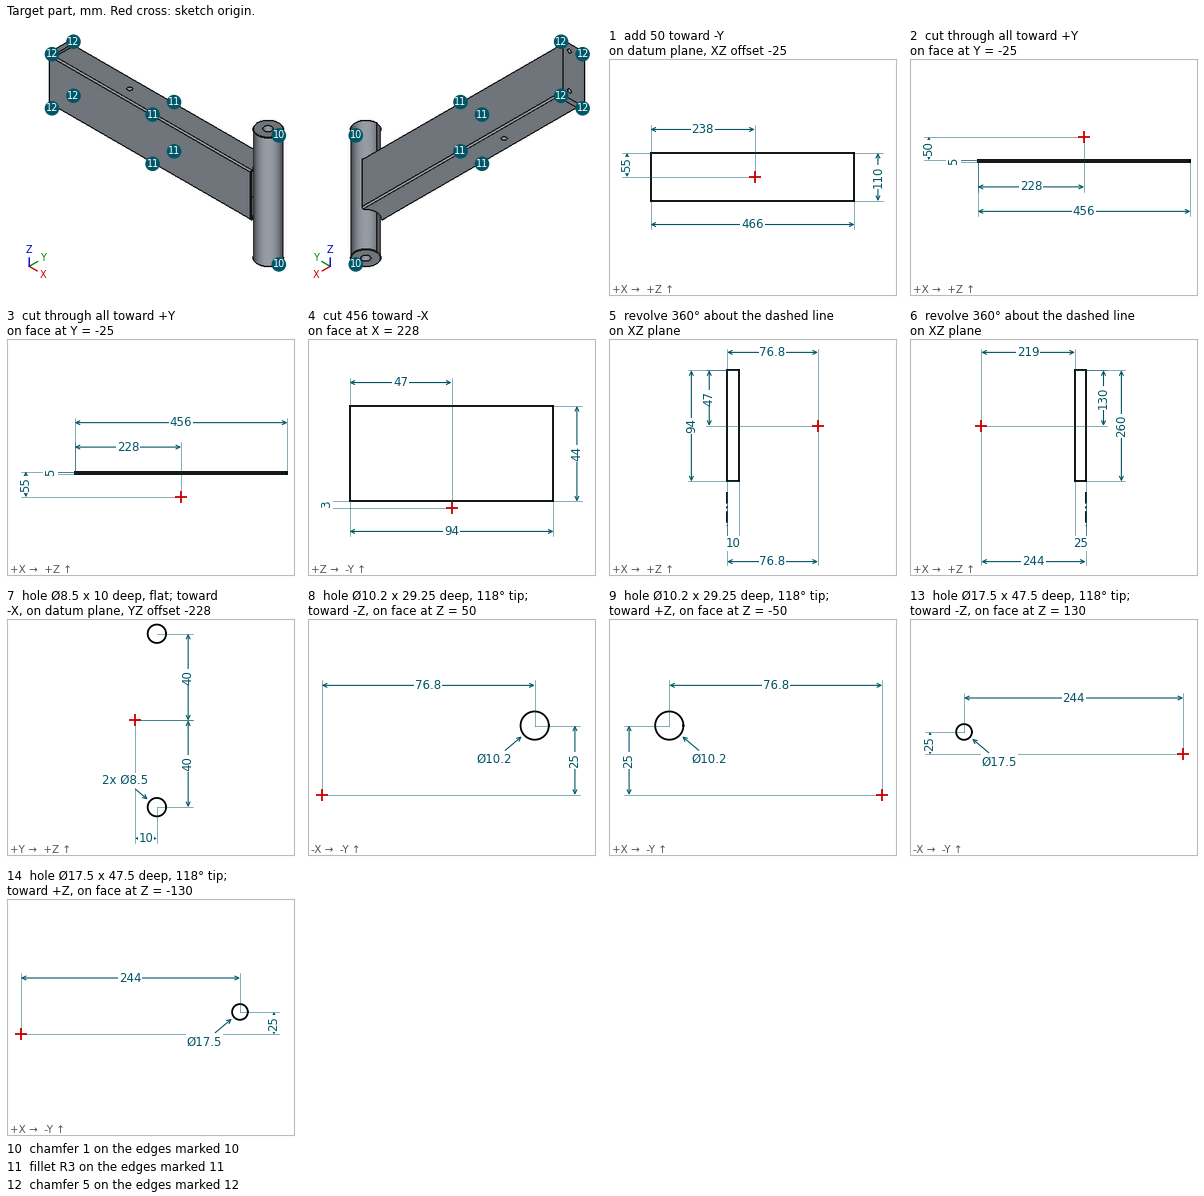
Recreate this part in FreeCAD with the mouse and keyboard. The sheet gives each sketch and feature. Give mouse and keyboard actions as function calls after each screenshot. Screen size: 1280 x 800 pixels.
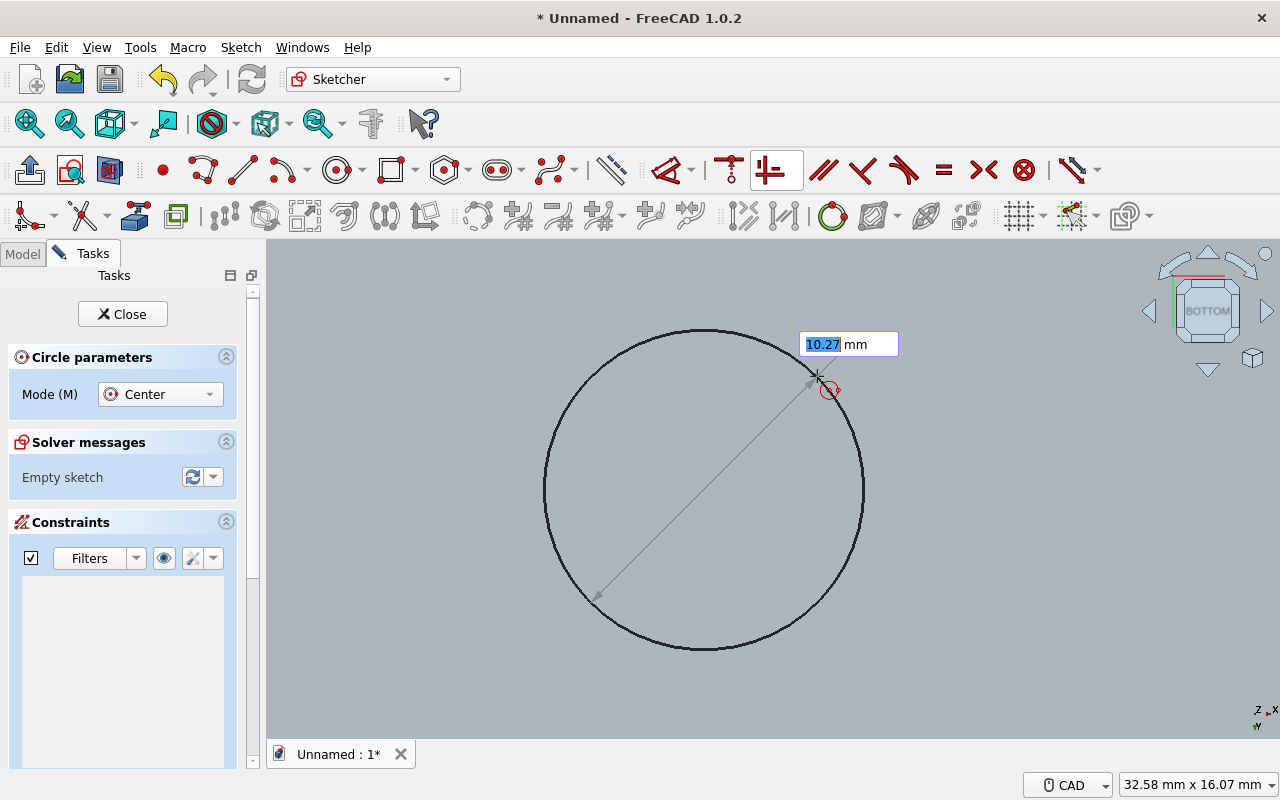
text(10.2)
key(Return)
key(Escape)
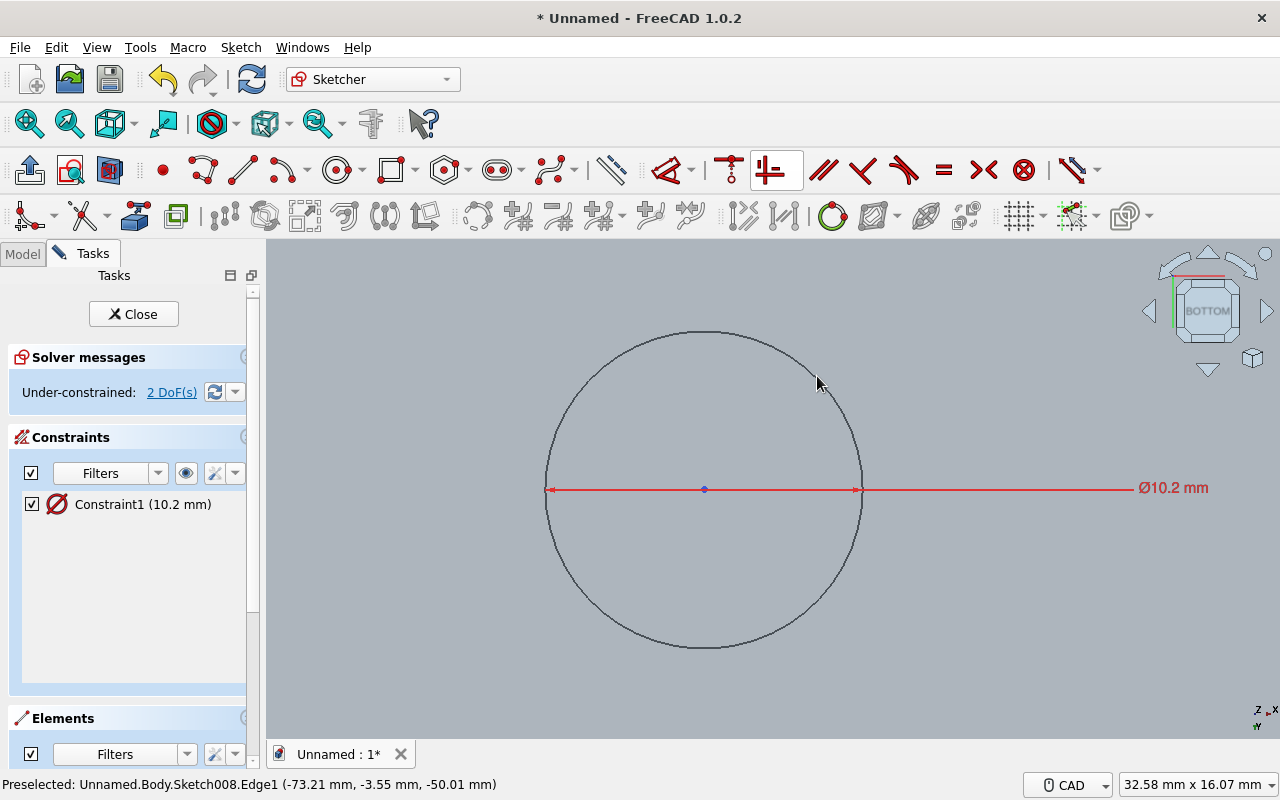
click(666, 170)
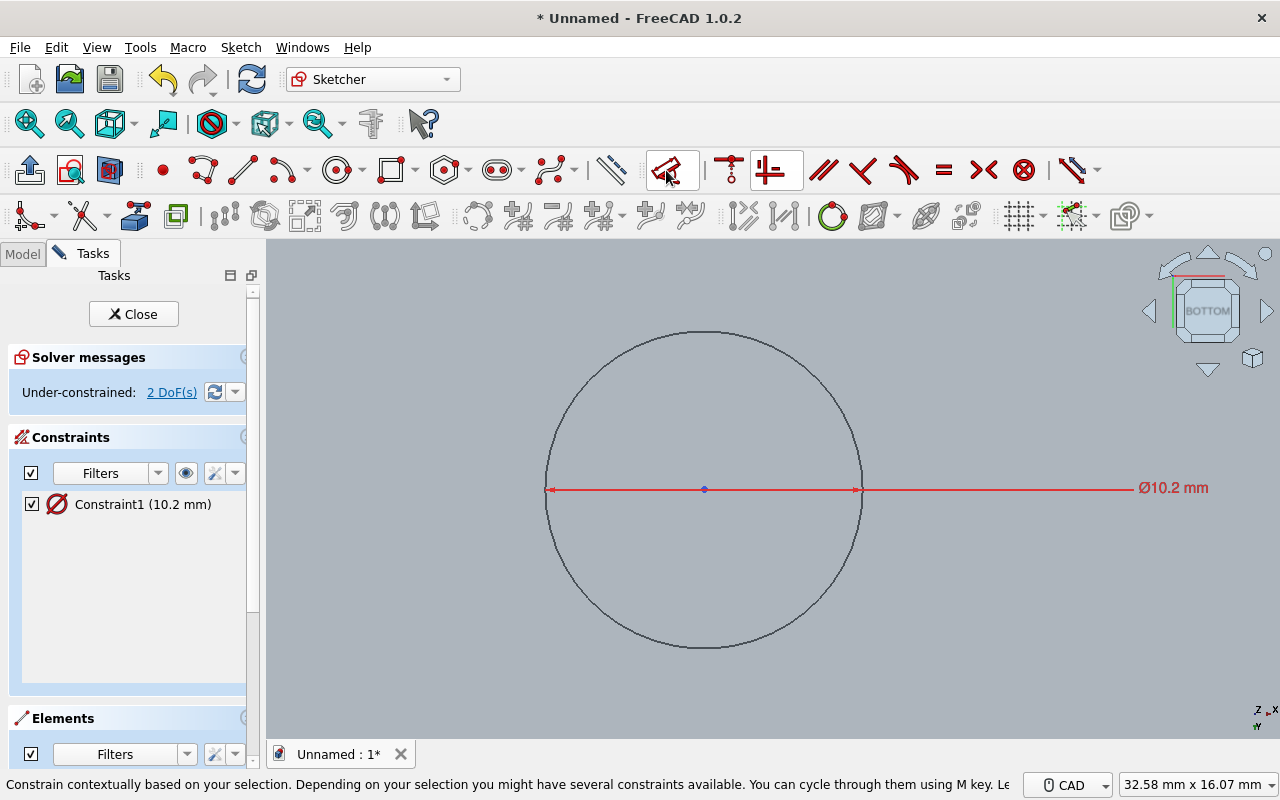
click(704, 490)
click(670, 601)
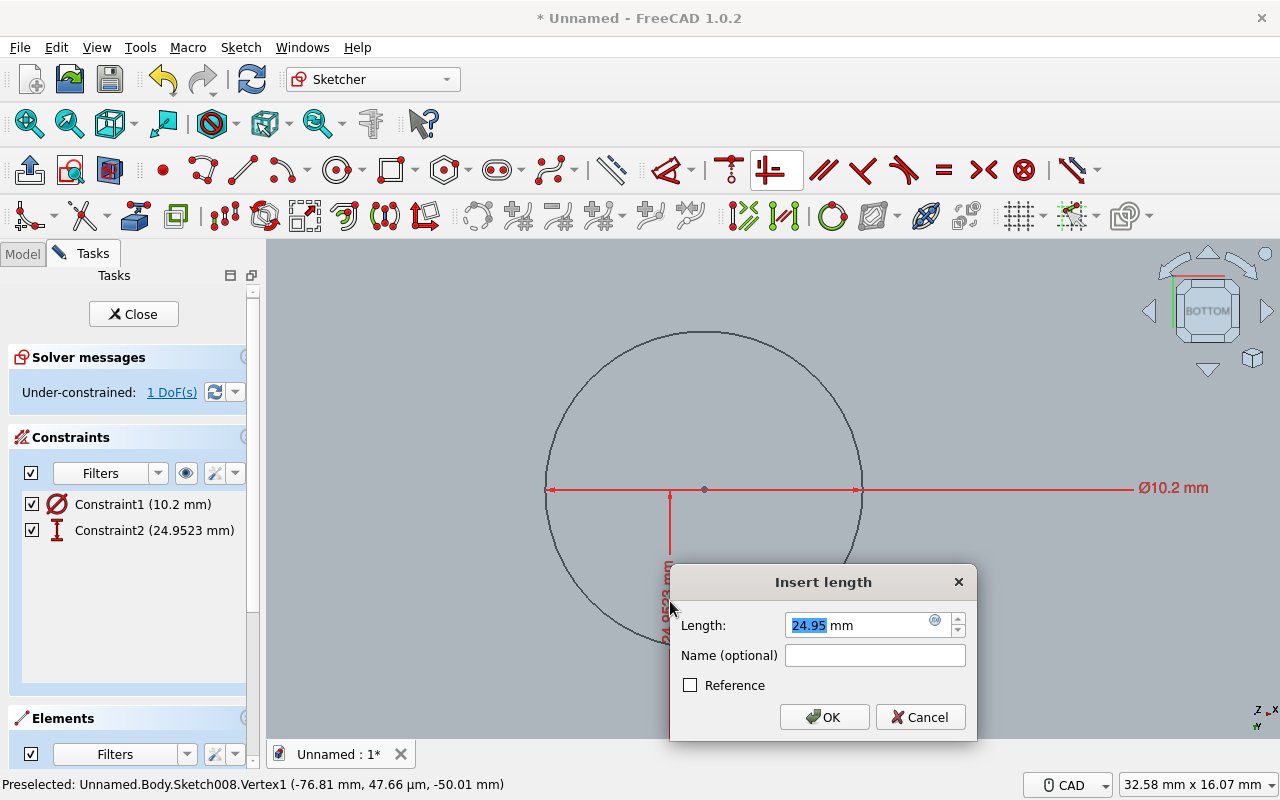
text(25)
key(Return)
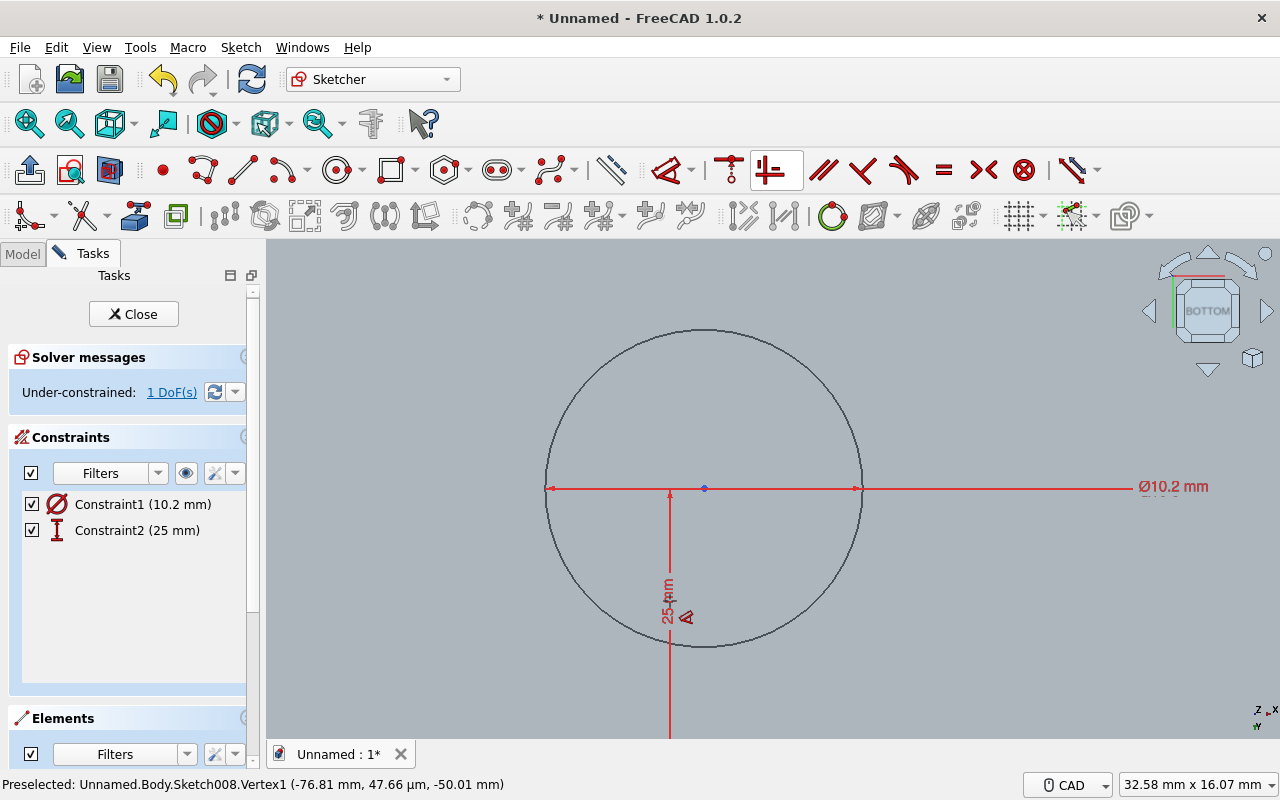
click(704, 489)
click(910, 455)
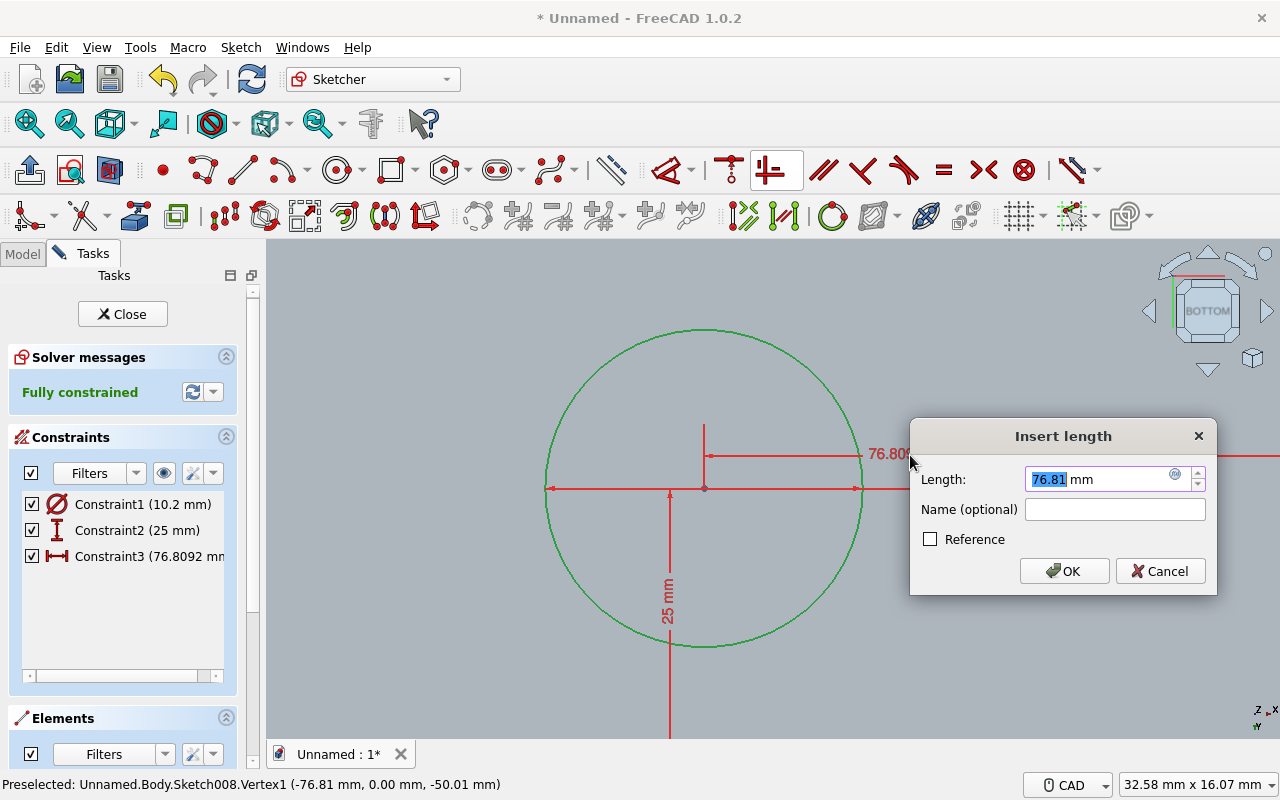
text(76.8)
key(Return)
key(Escape)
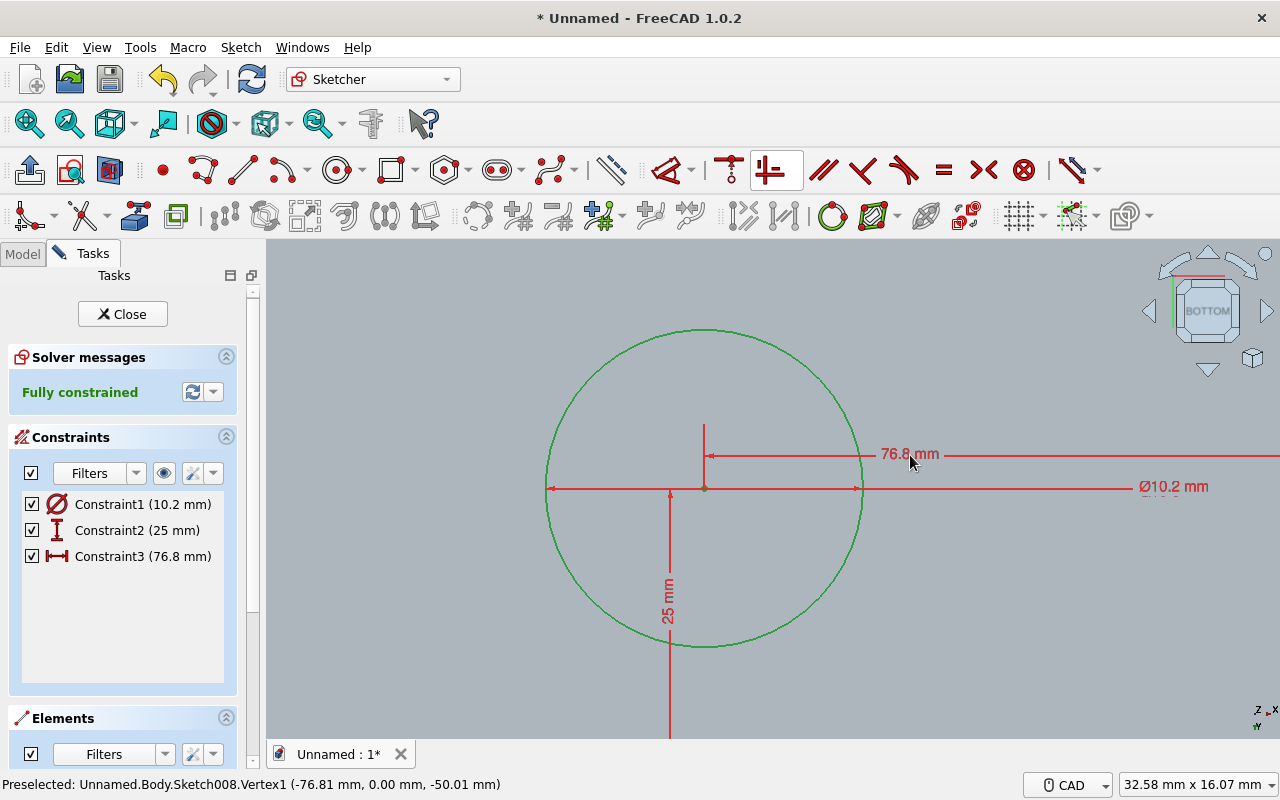
click(123, 314)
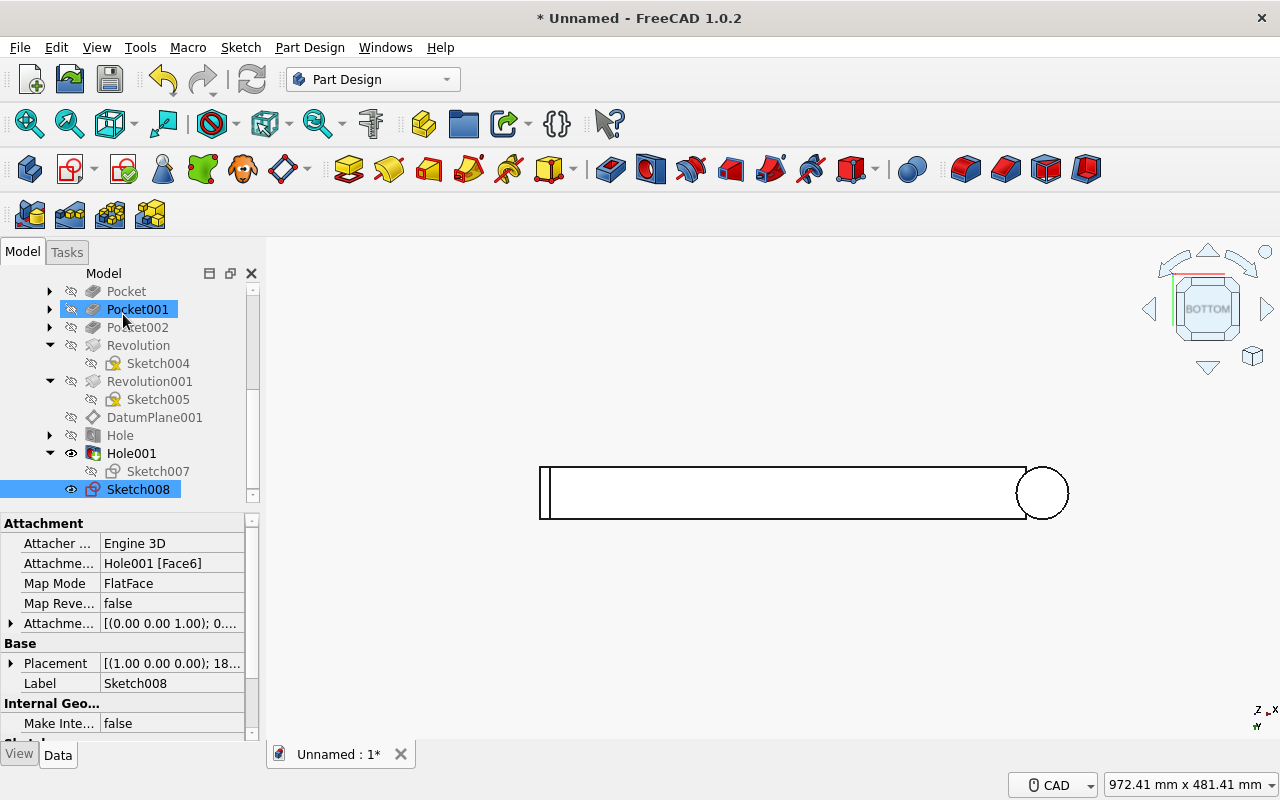
click(652, 170)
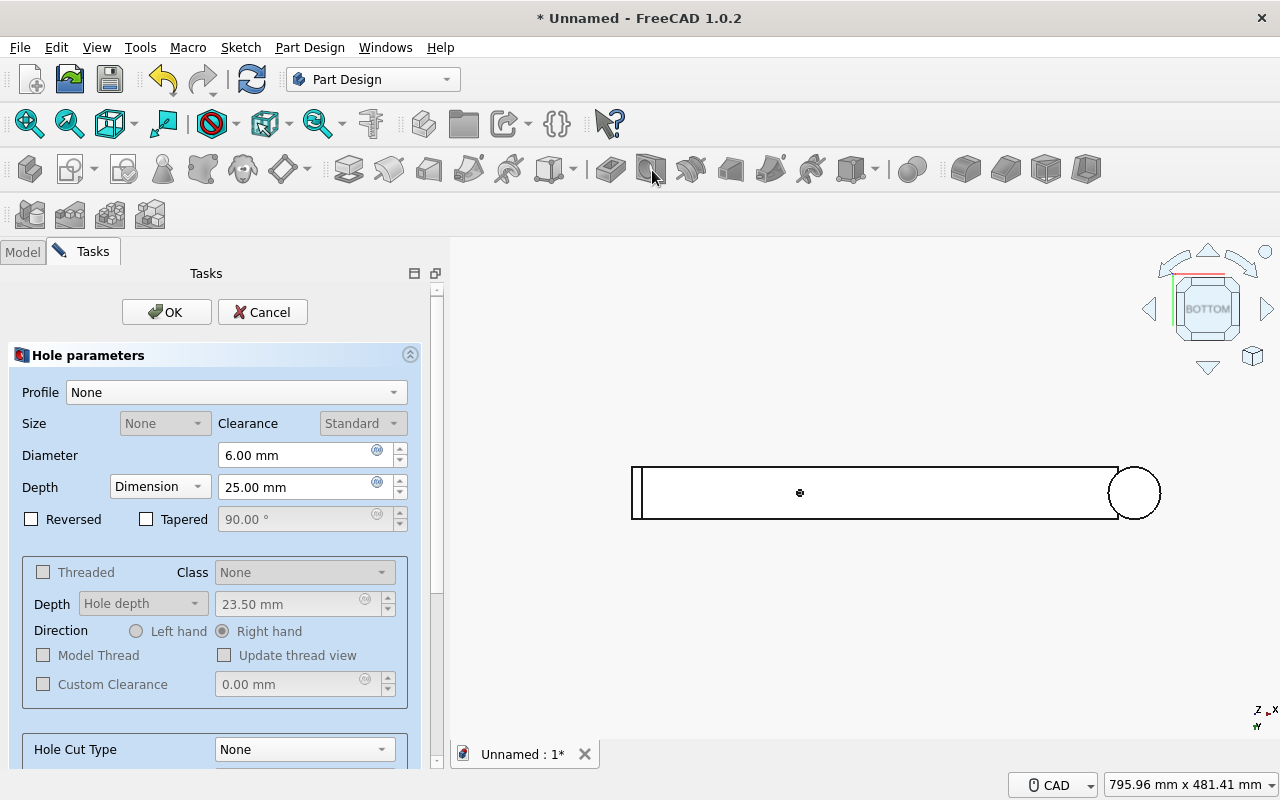
triple_click(305, 455)